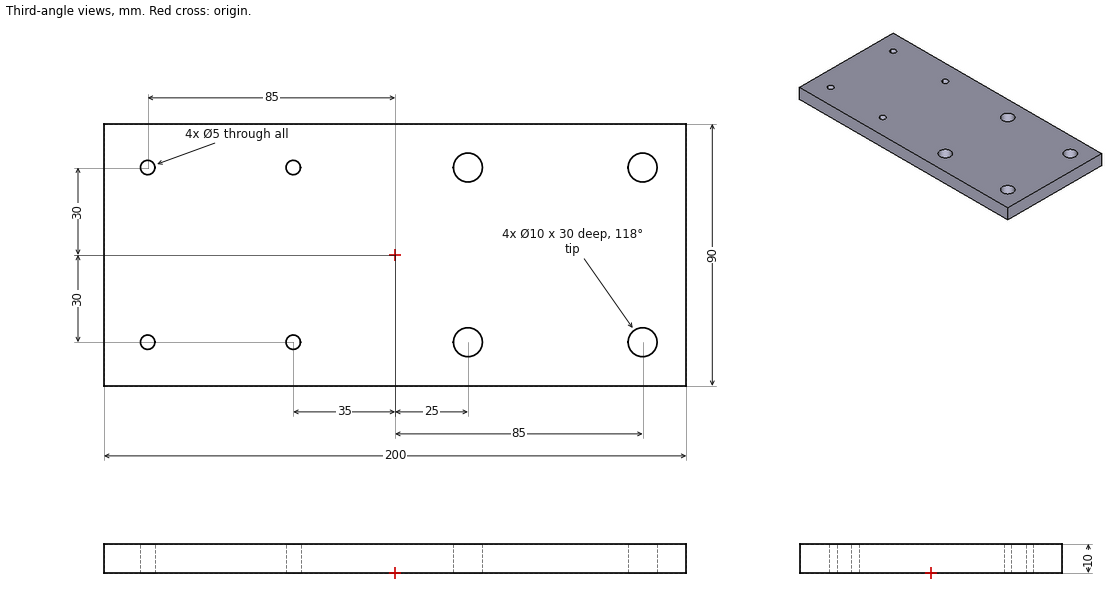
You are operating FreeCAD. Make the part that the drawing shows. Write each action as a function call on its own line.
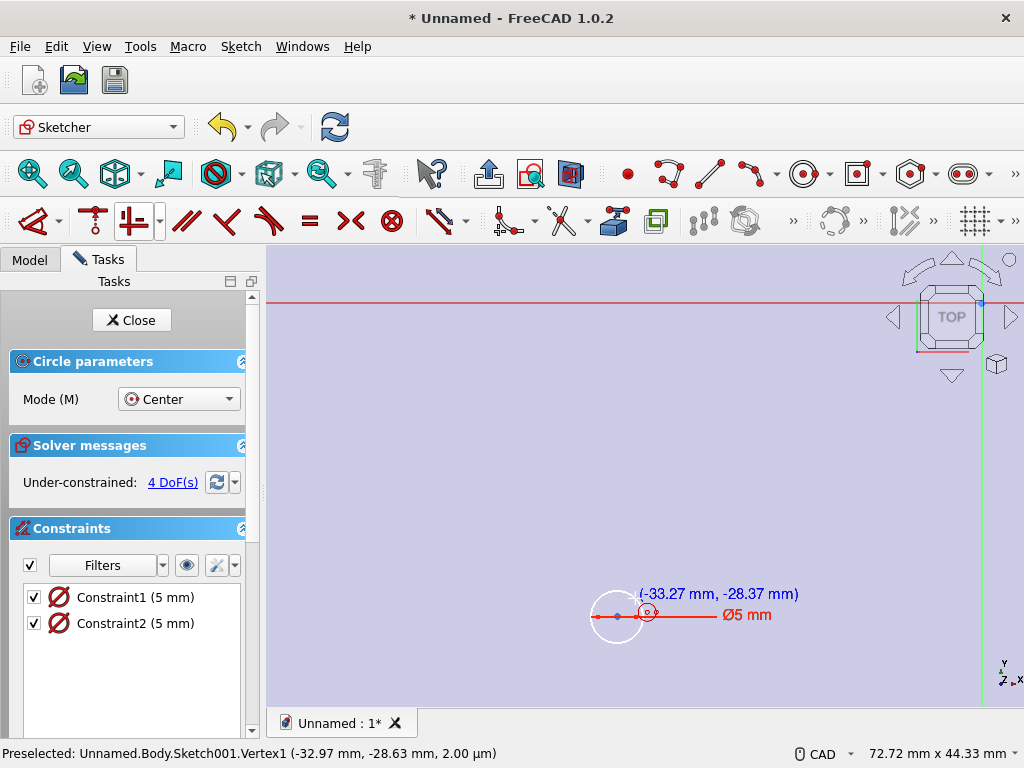
scroll(618, 617, down, 4)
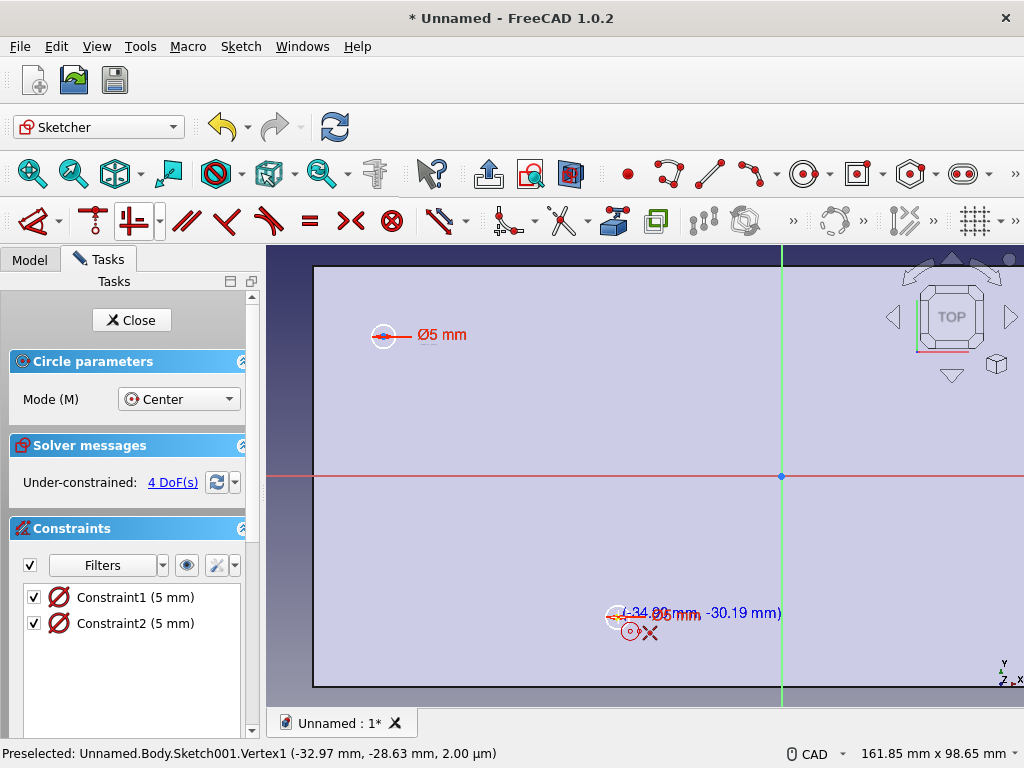
scroll(384, 617, up, 4)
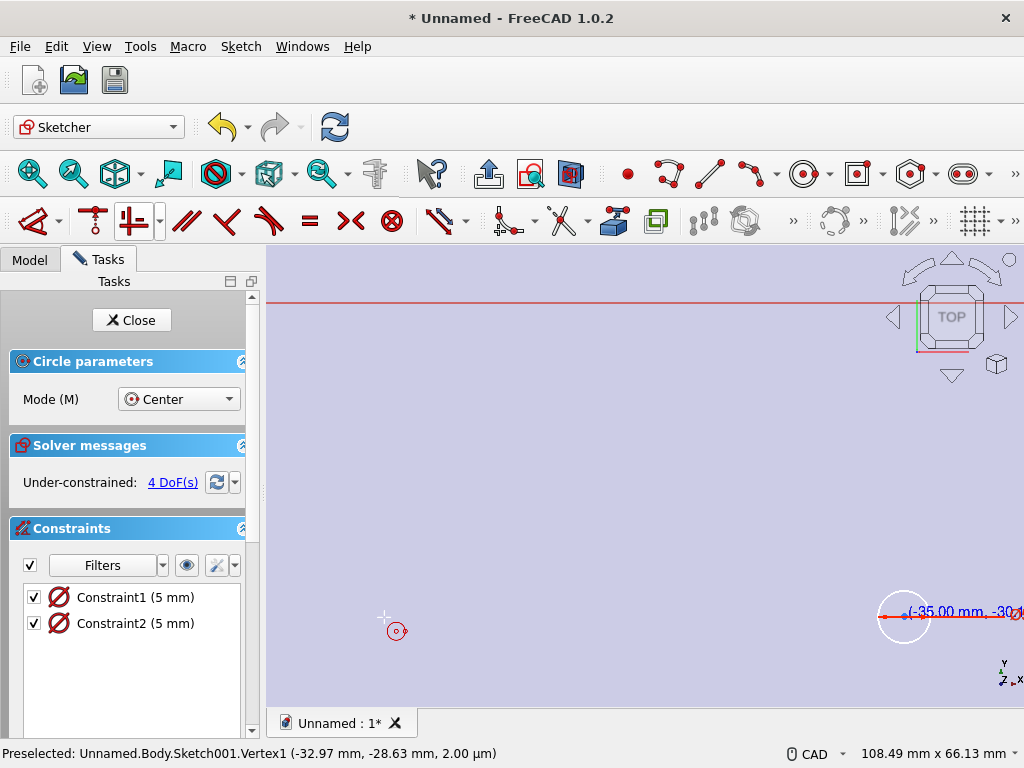
click(383, 616)
move(401, 598)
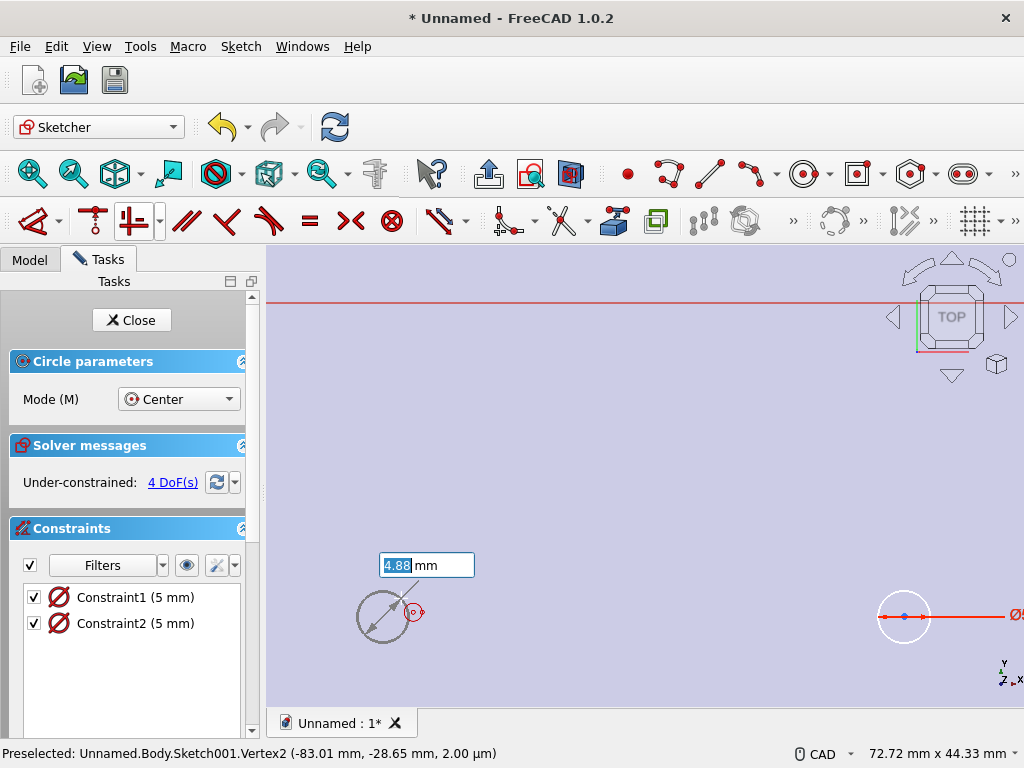
text(5)
key(Return)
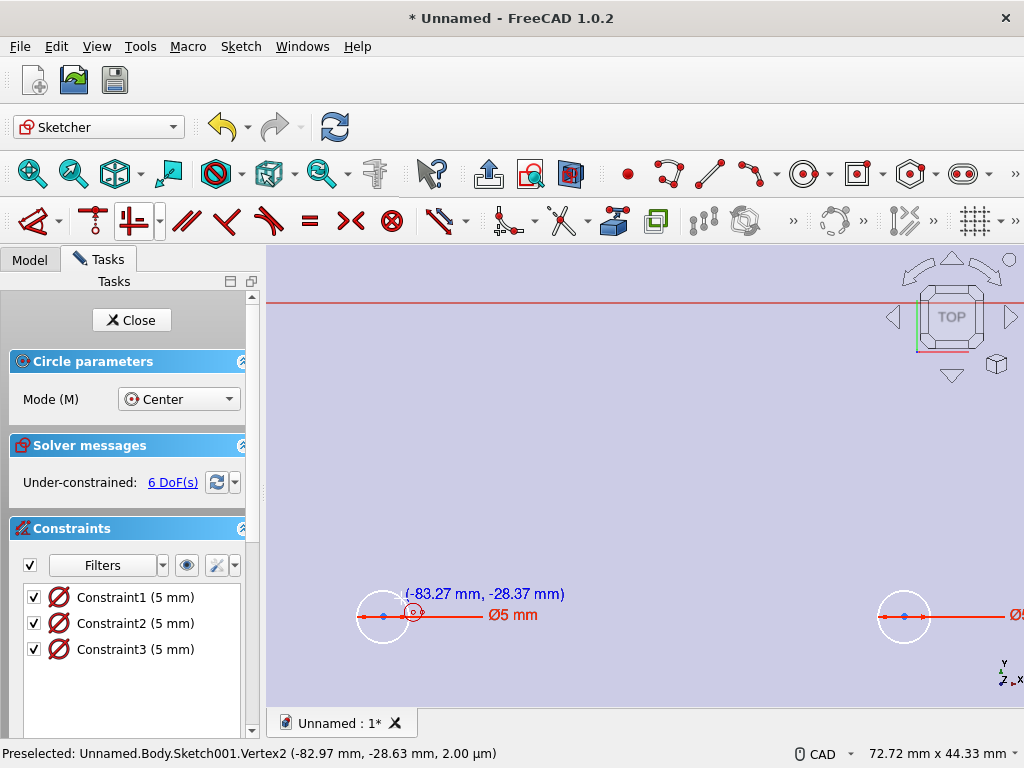
scroll(384, 617, down, 4)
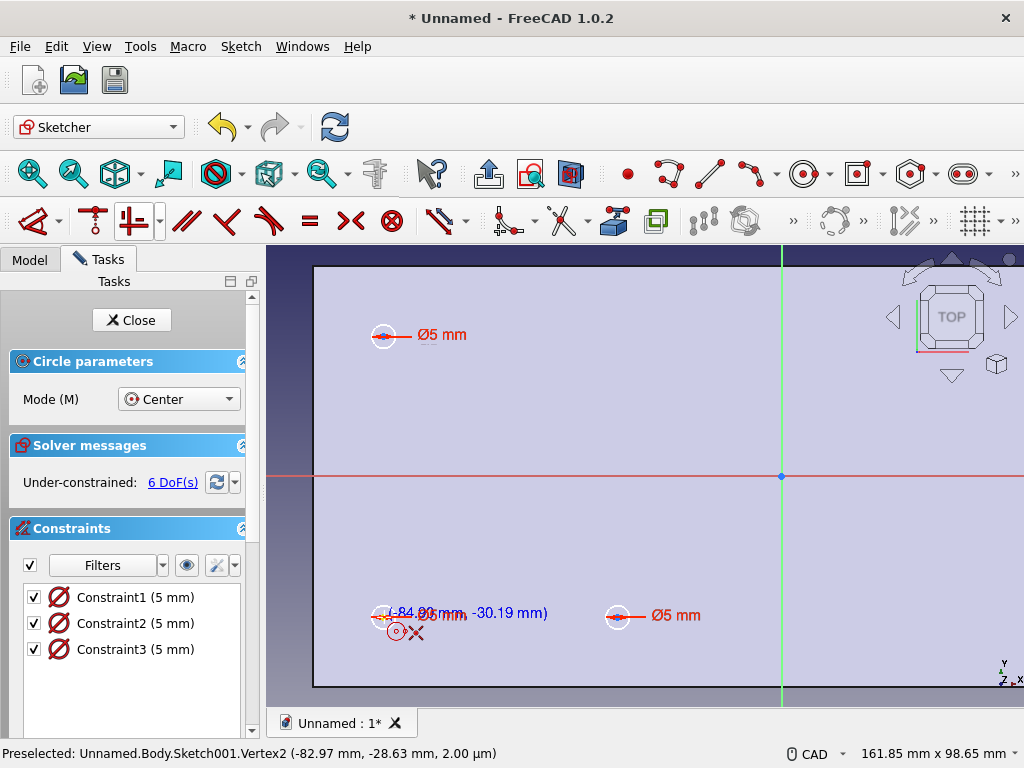
scroll(618, 336, up, 4)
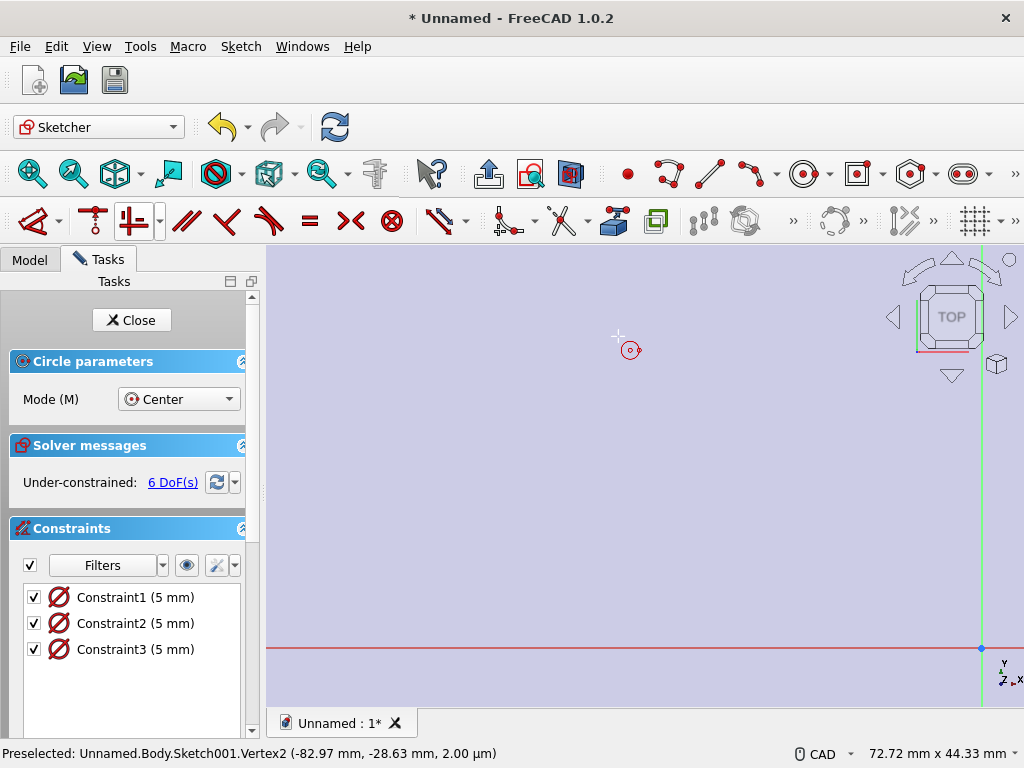
click(617, 336)
move(635, 317)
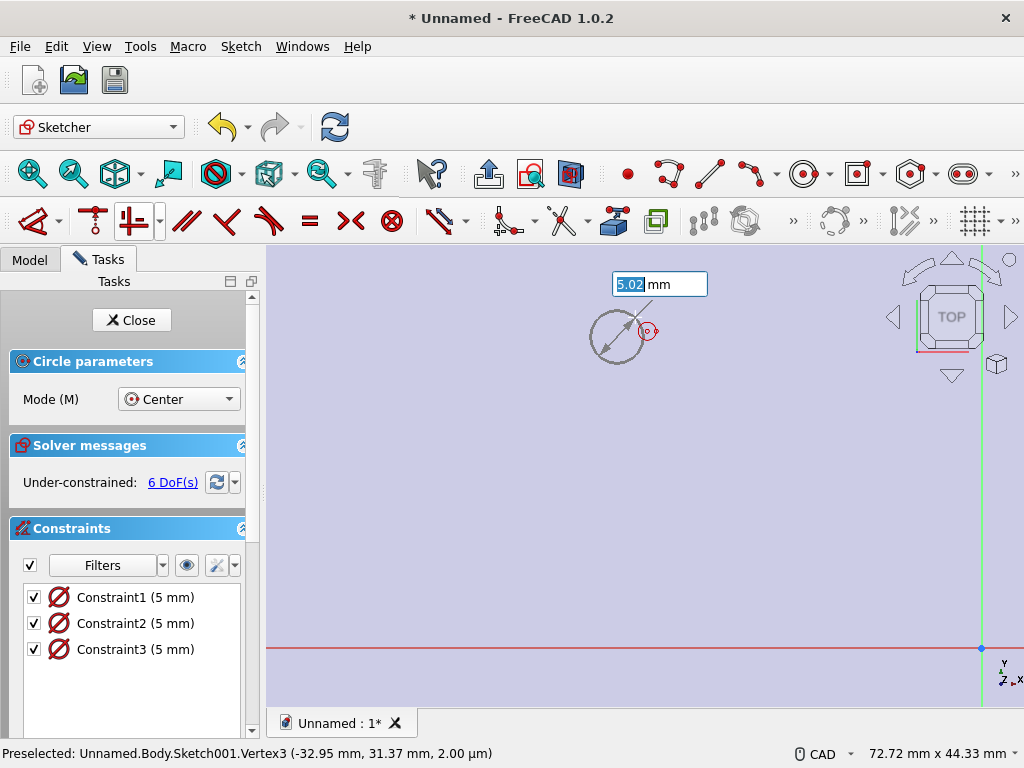
text(5)
key(Return)
key(Escape)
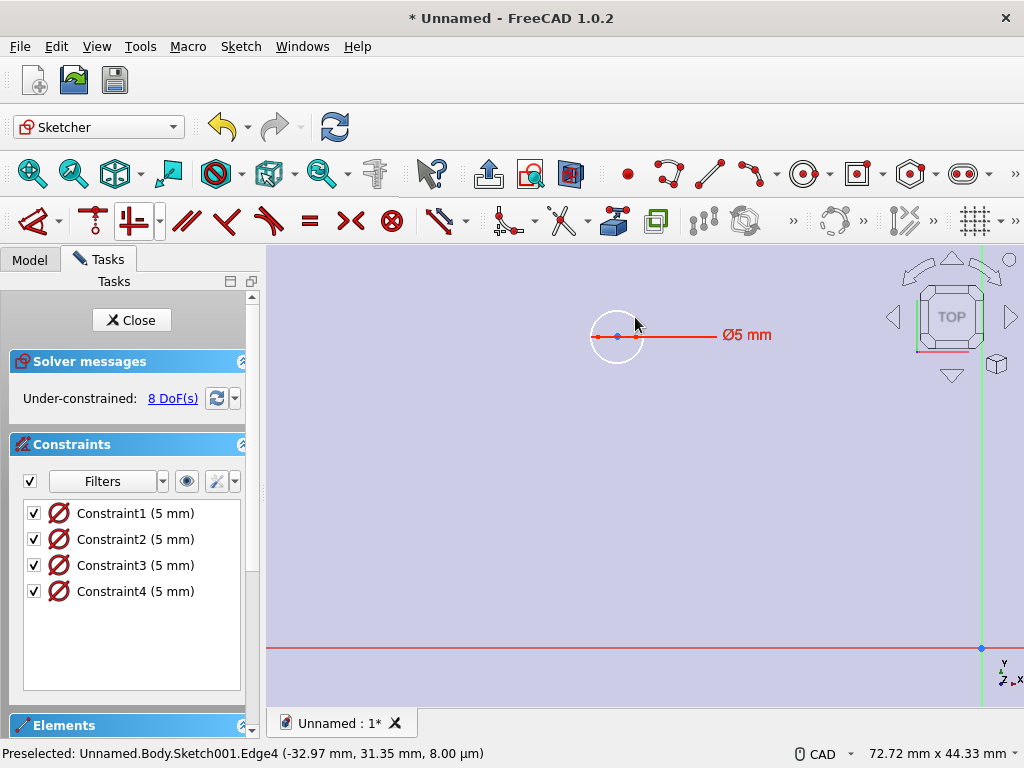
scroll(618, 335, down, 4)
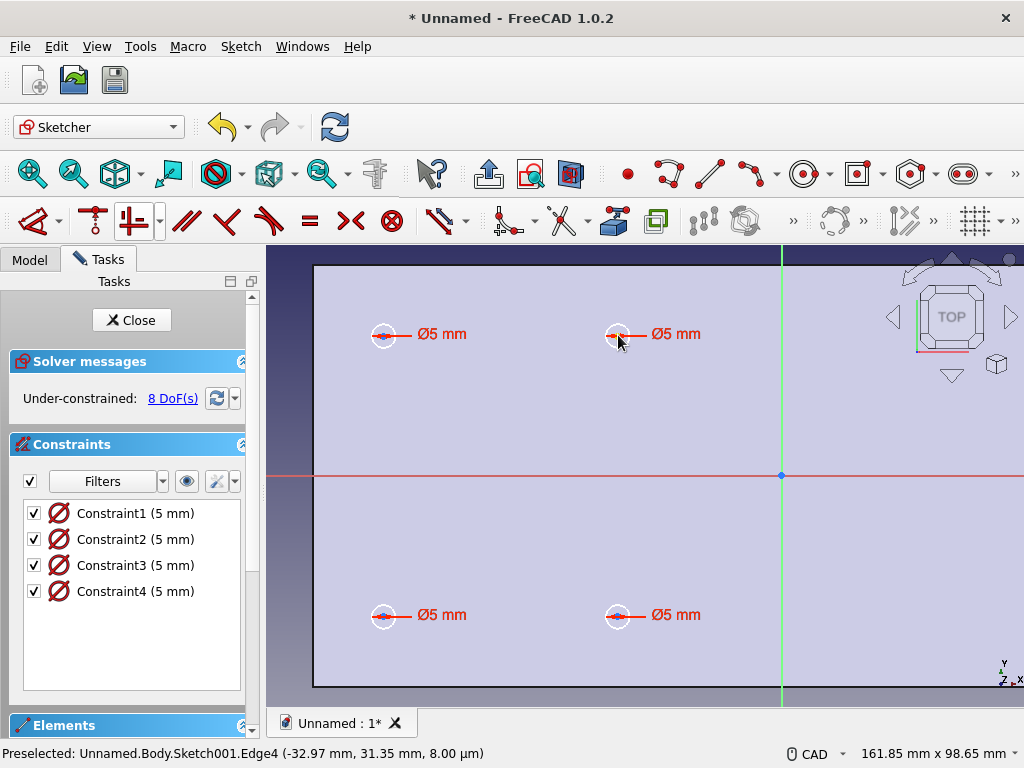
click(384, 336)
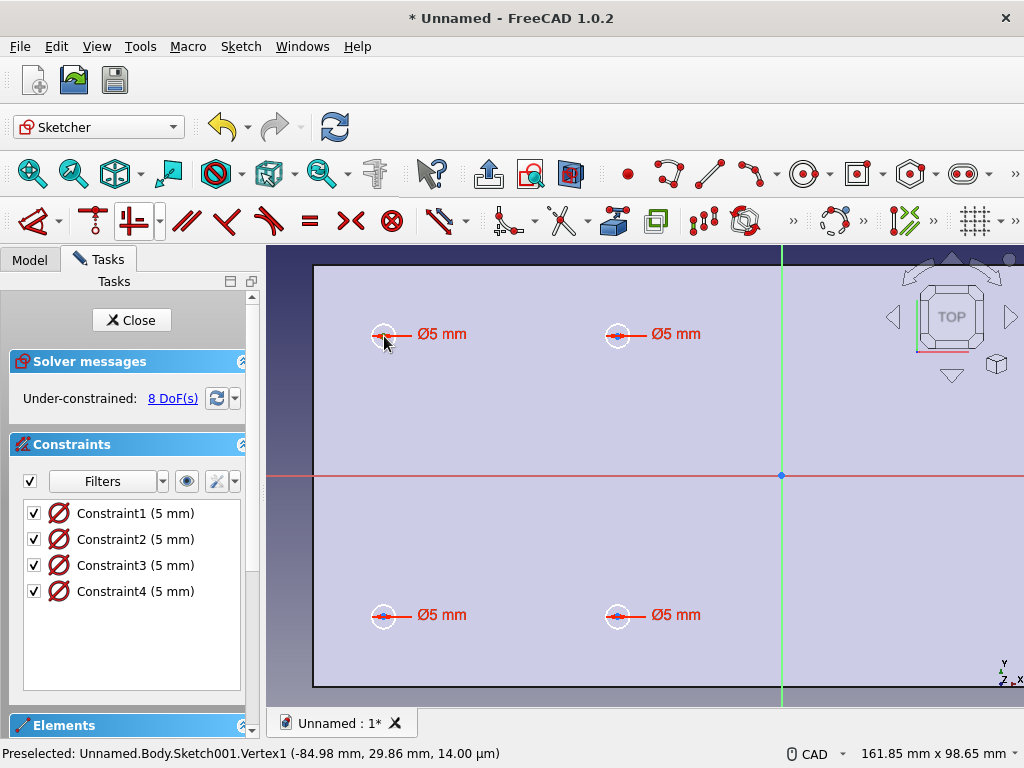
click(384, 617)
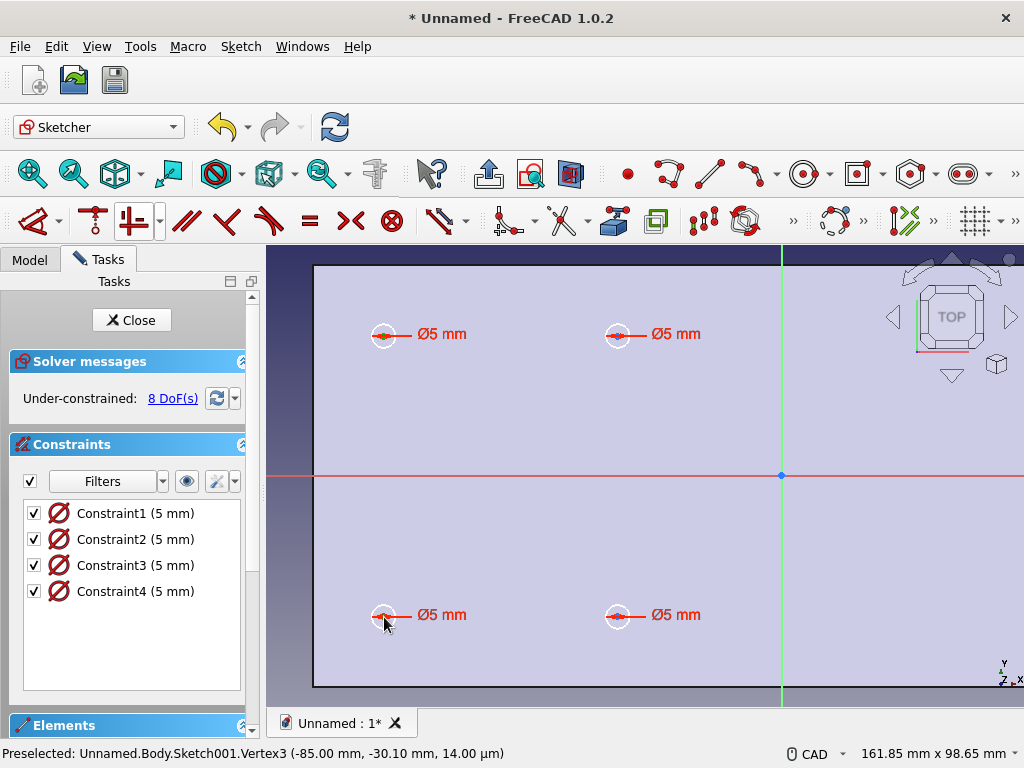
key(v)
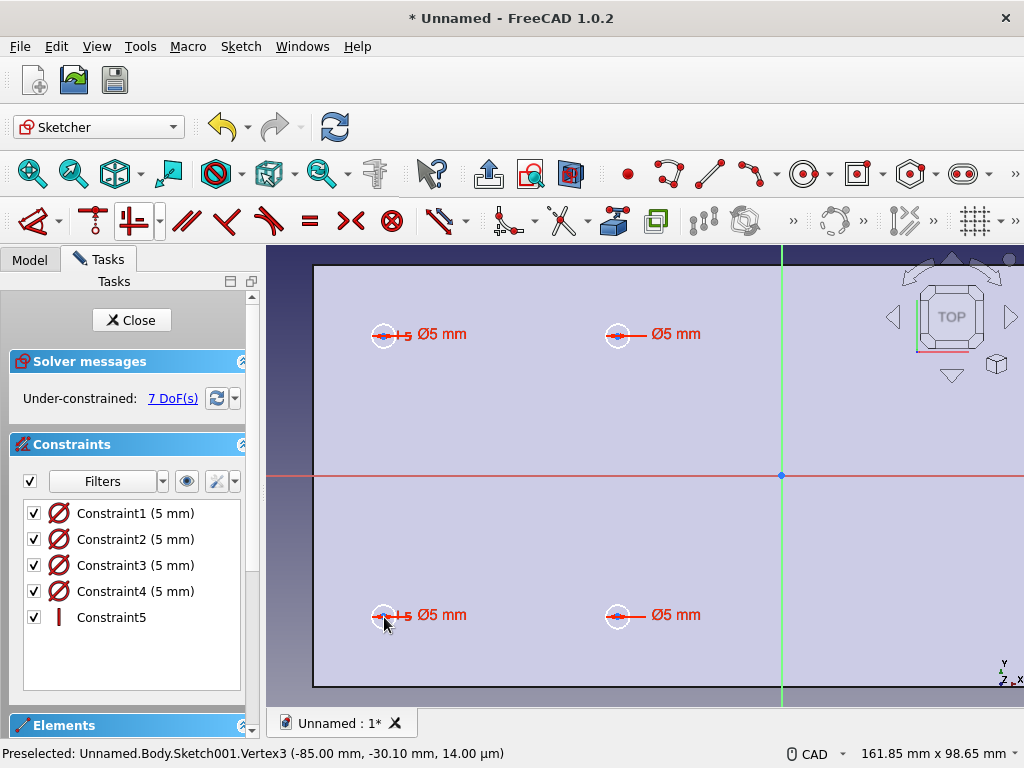
click(618, 617)